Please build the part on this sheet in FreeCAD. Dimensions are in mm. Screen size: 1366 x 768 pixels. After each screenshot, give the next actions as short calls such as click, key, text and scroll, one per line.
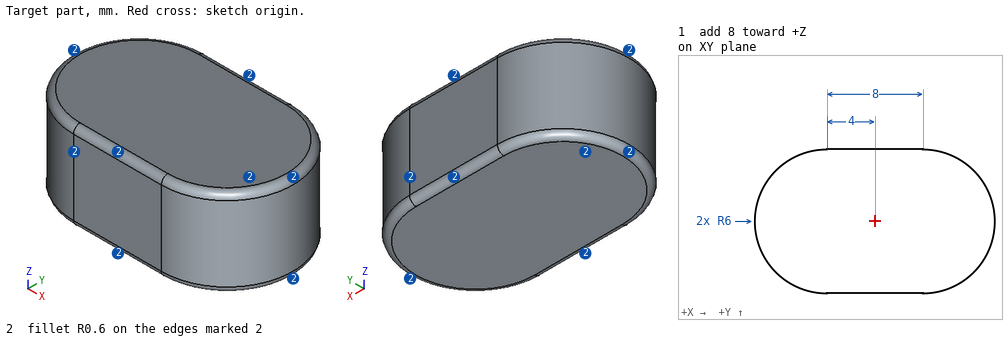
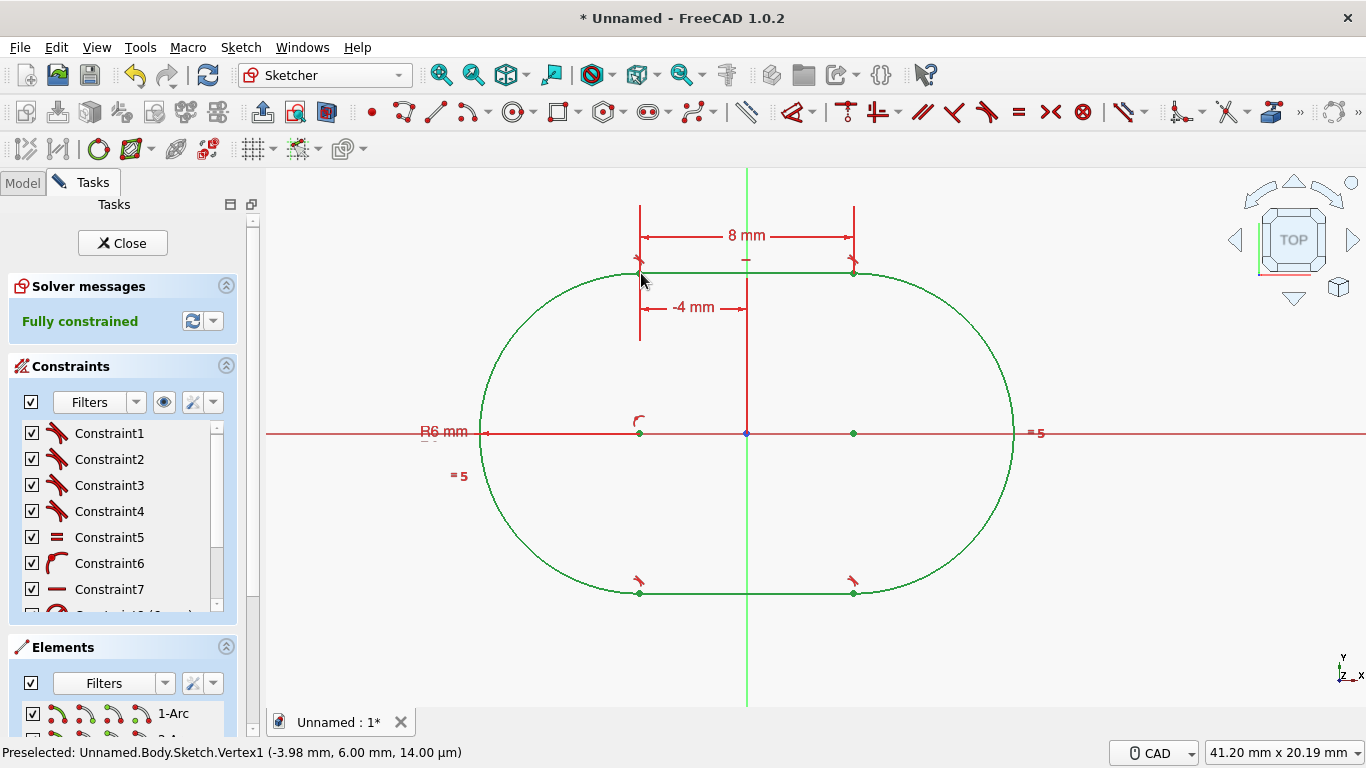
click(123, 243)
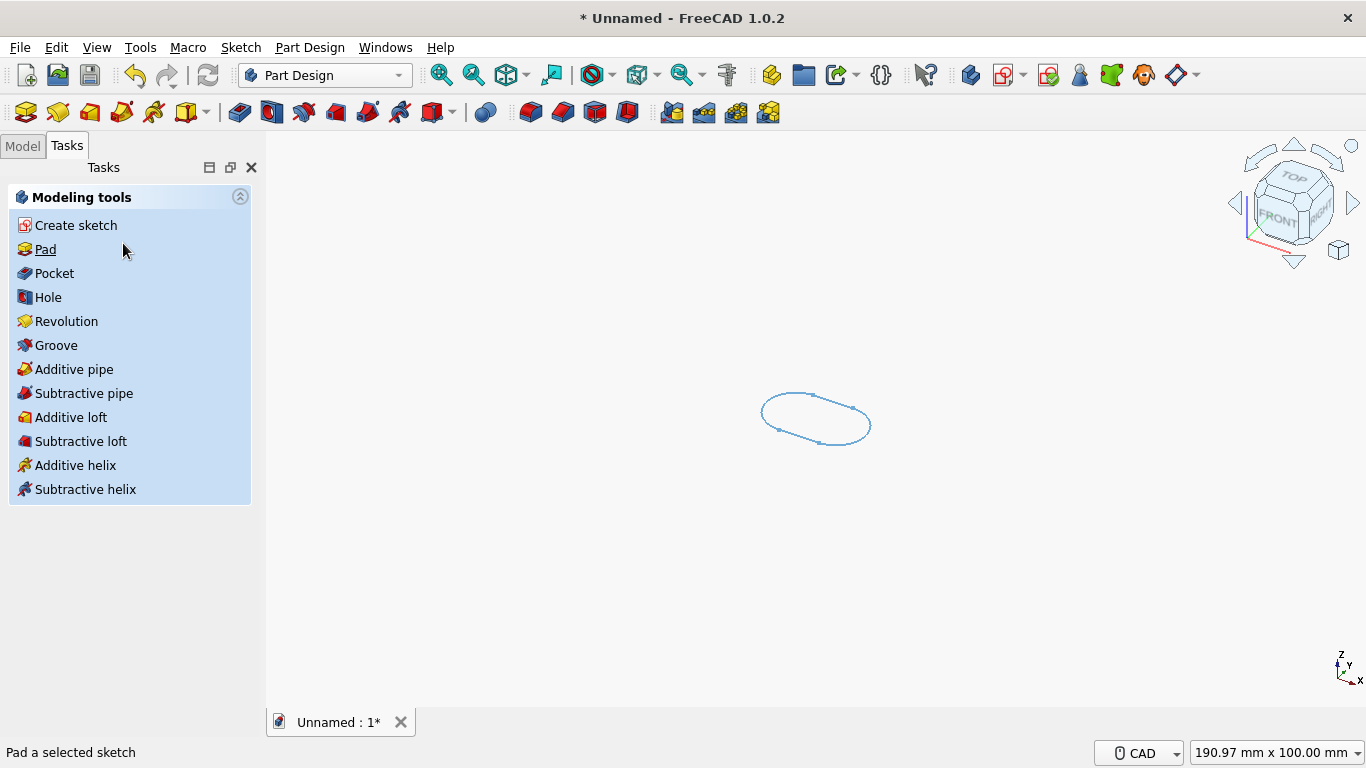
click(26, 112)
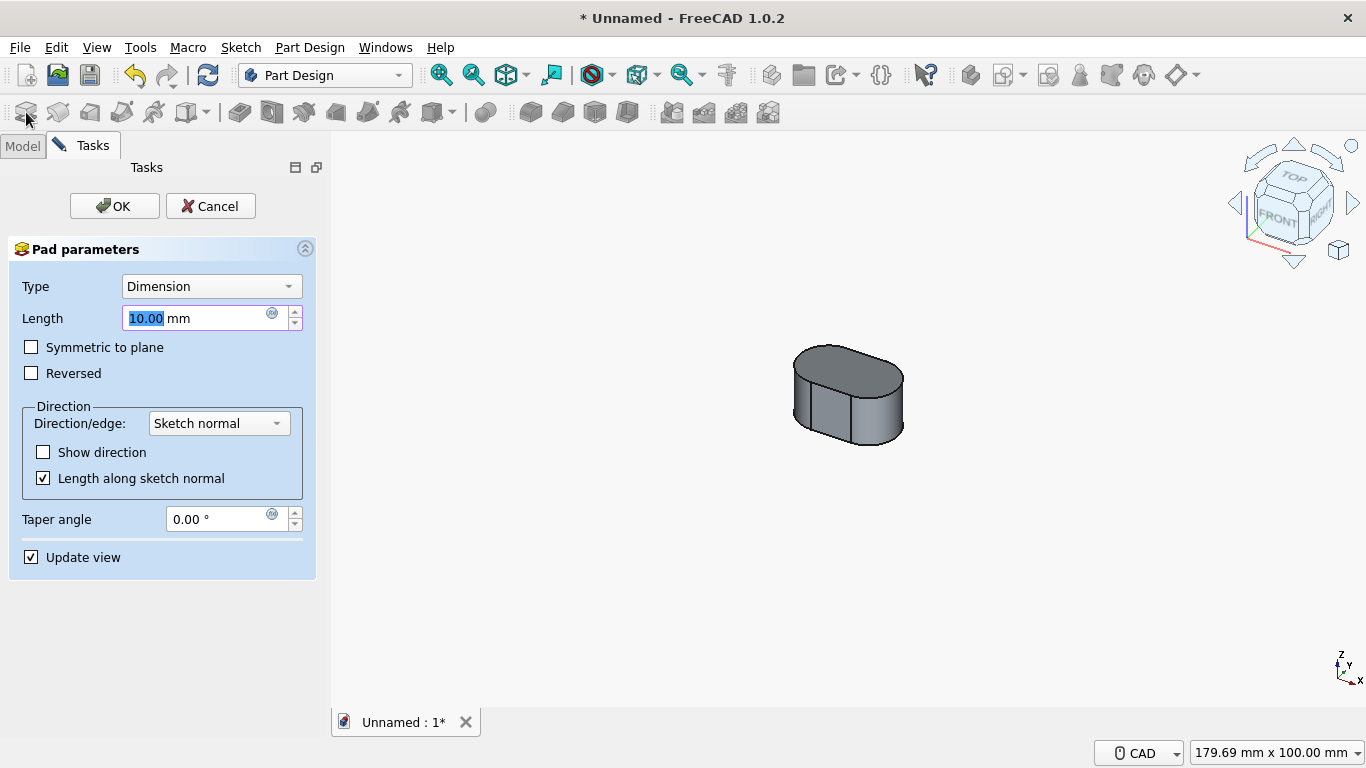
text(8)
key(Tab)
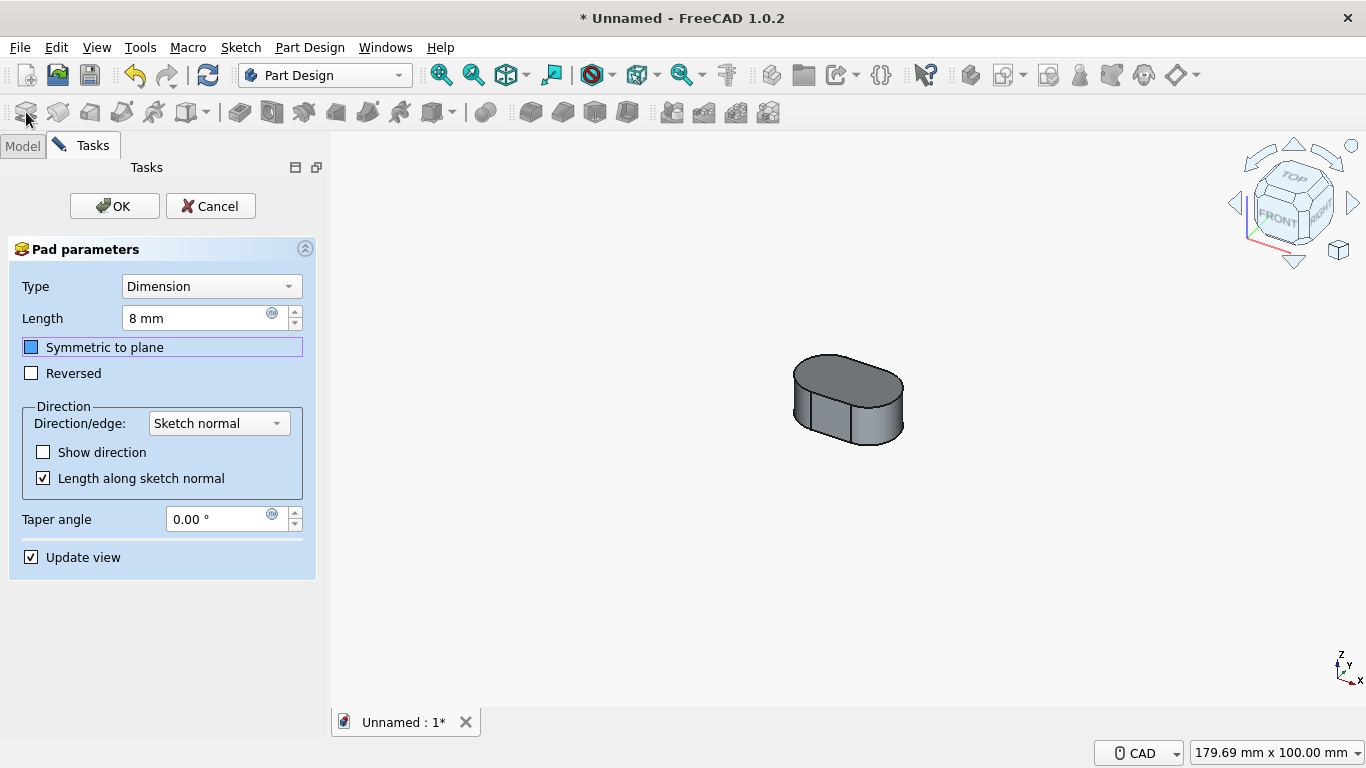
click(115, 206)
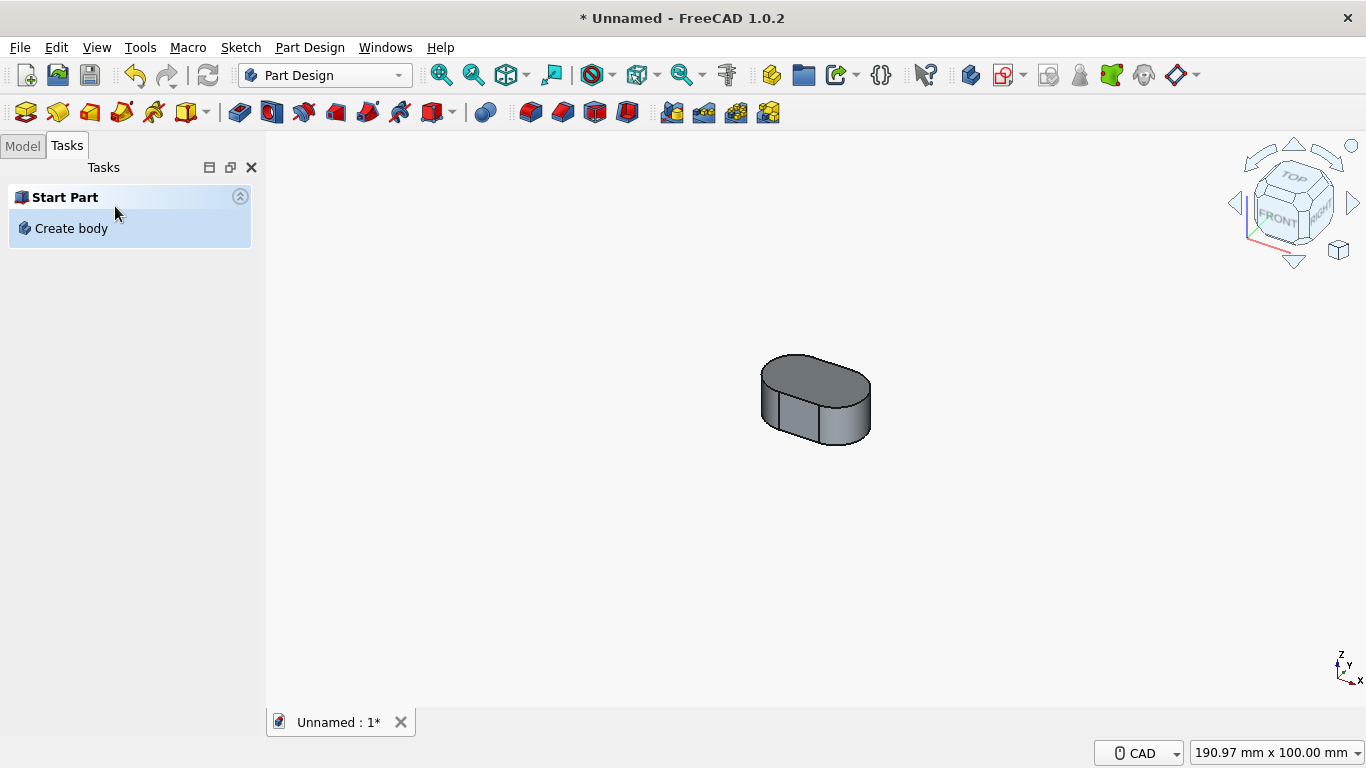
key(v)
key(f)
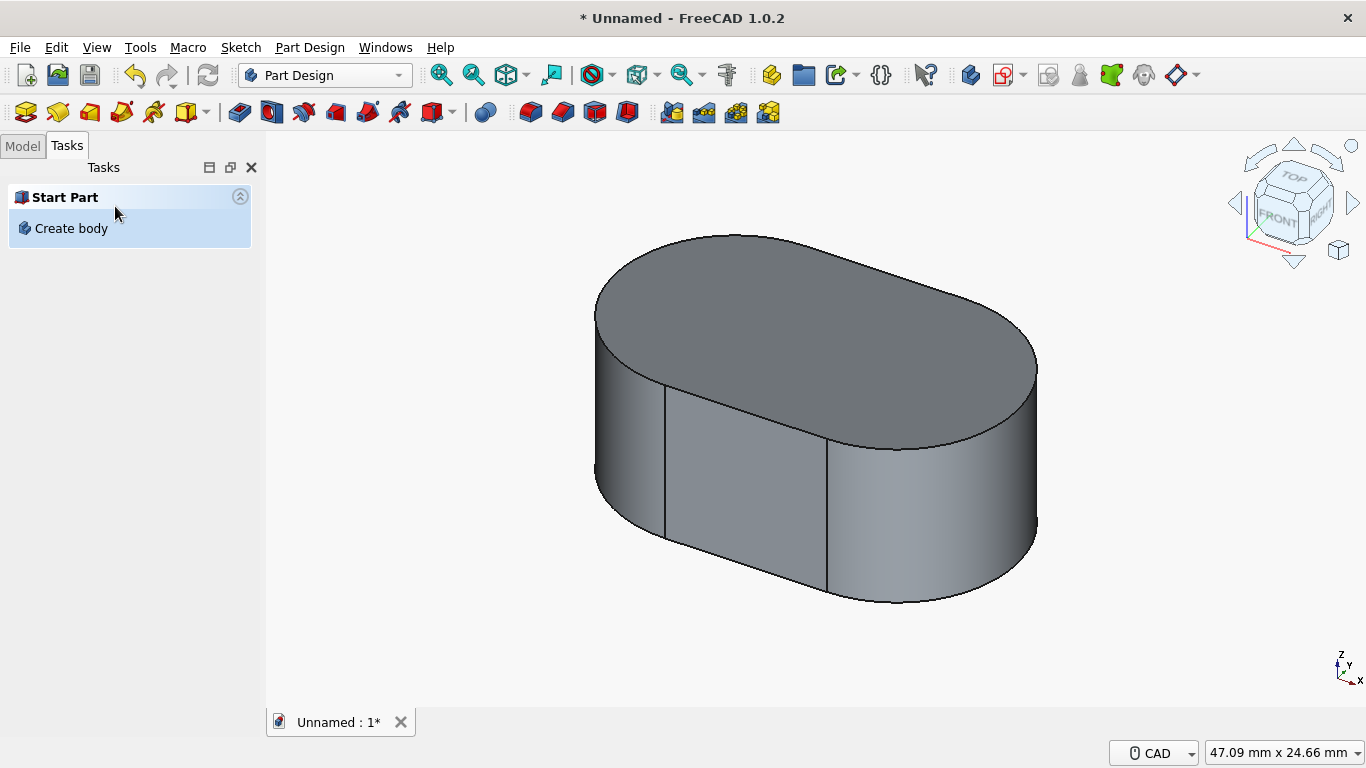
click(874, 361)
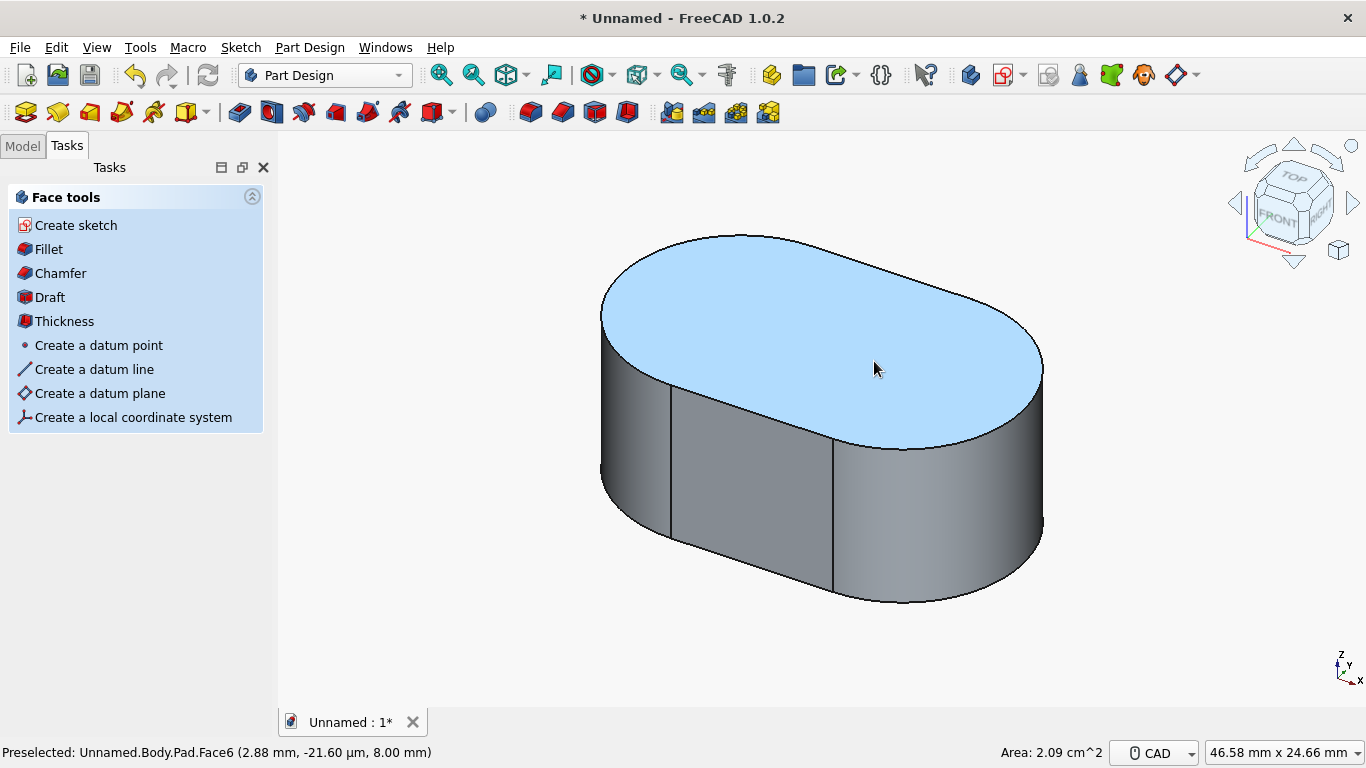
key(0)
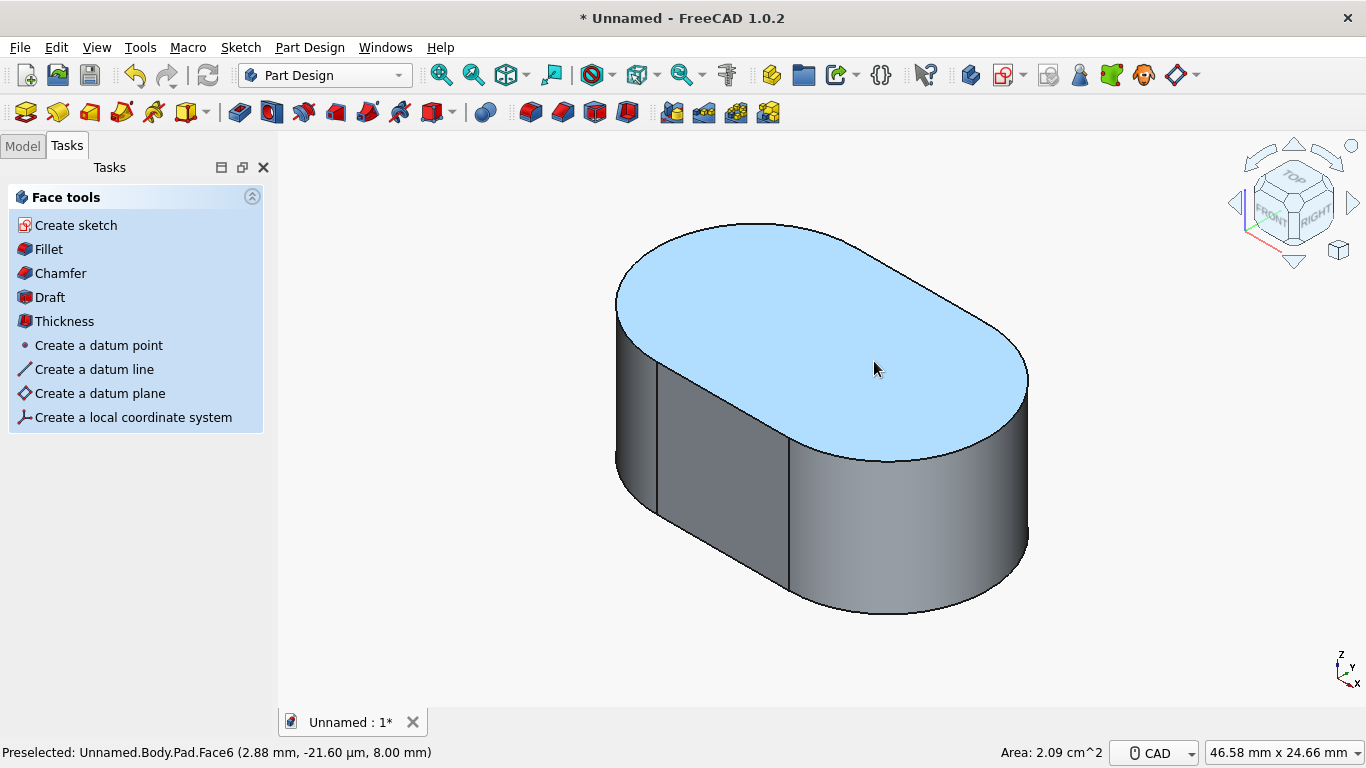
key(2)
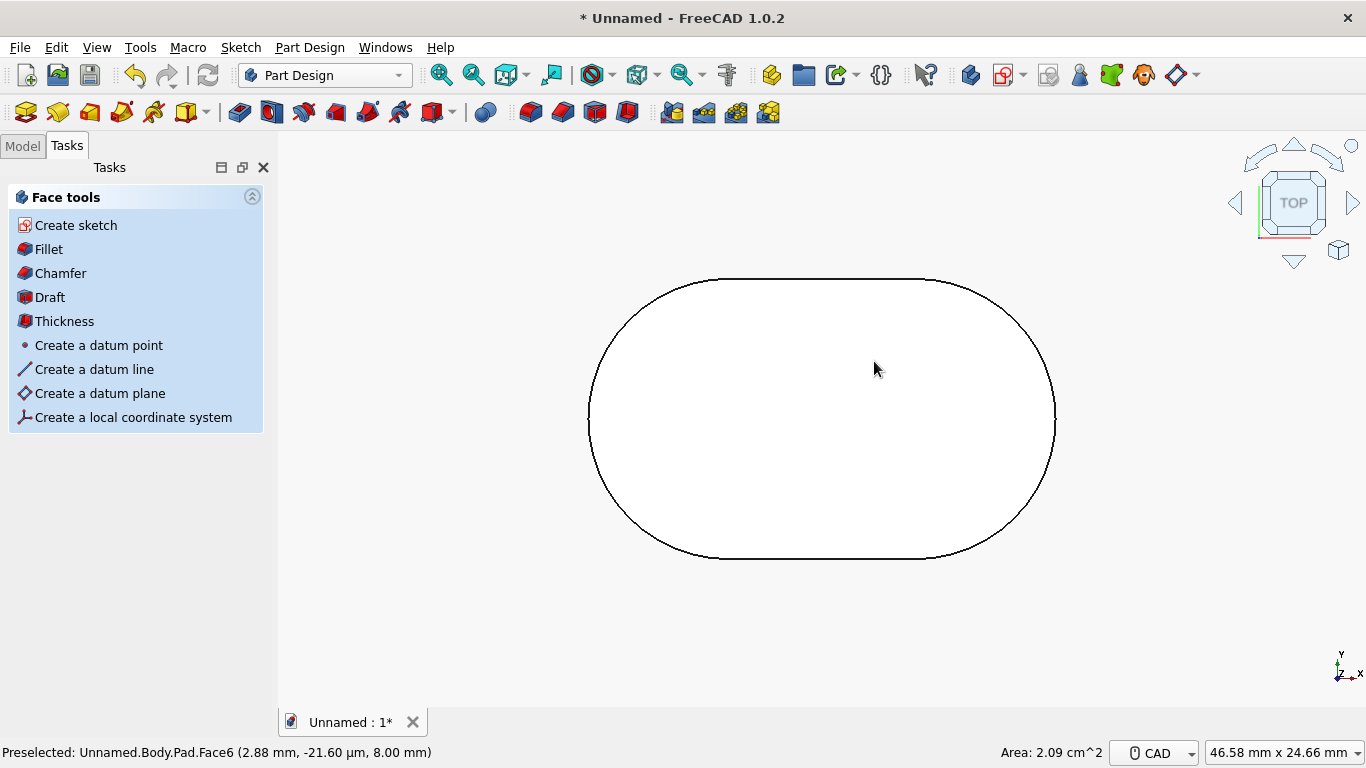
key(1)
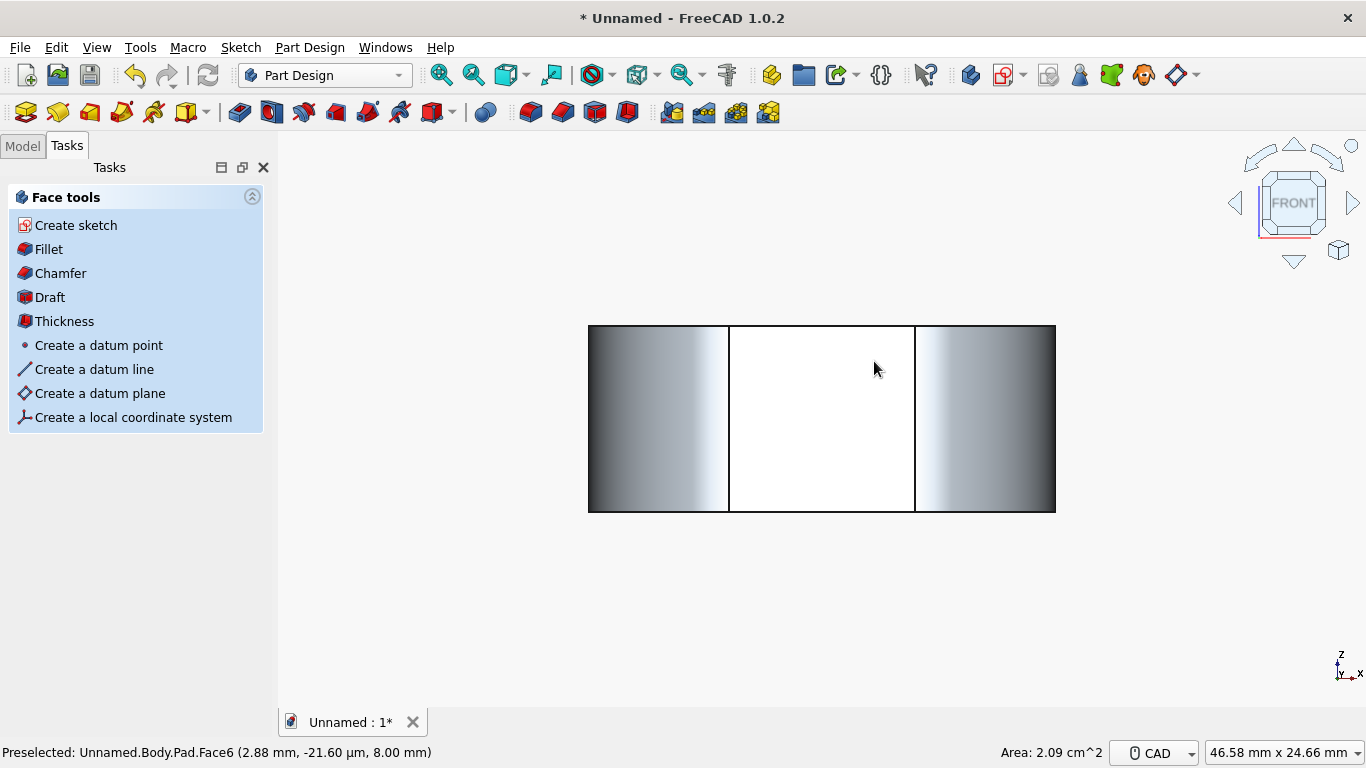
click(442, 76)